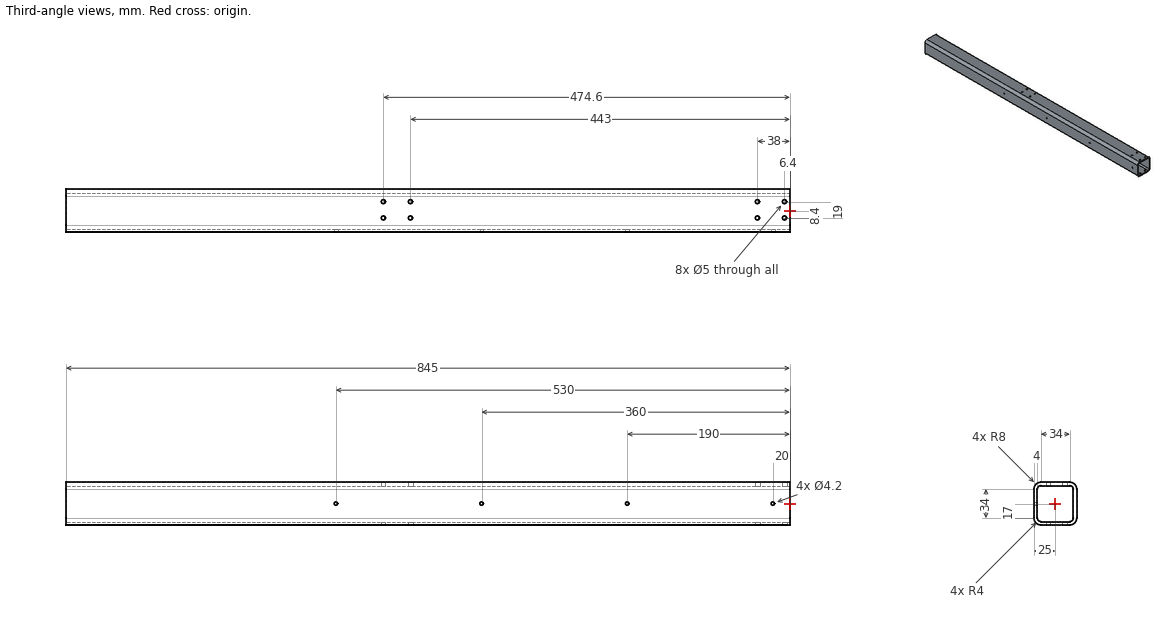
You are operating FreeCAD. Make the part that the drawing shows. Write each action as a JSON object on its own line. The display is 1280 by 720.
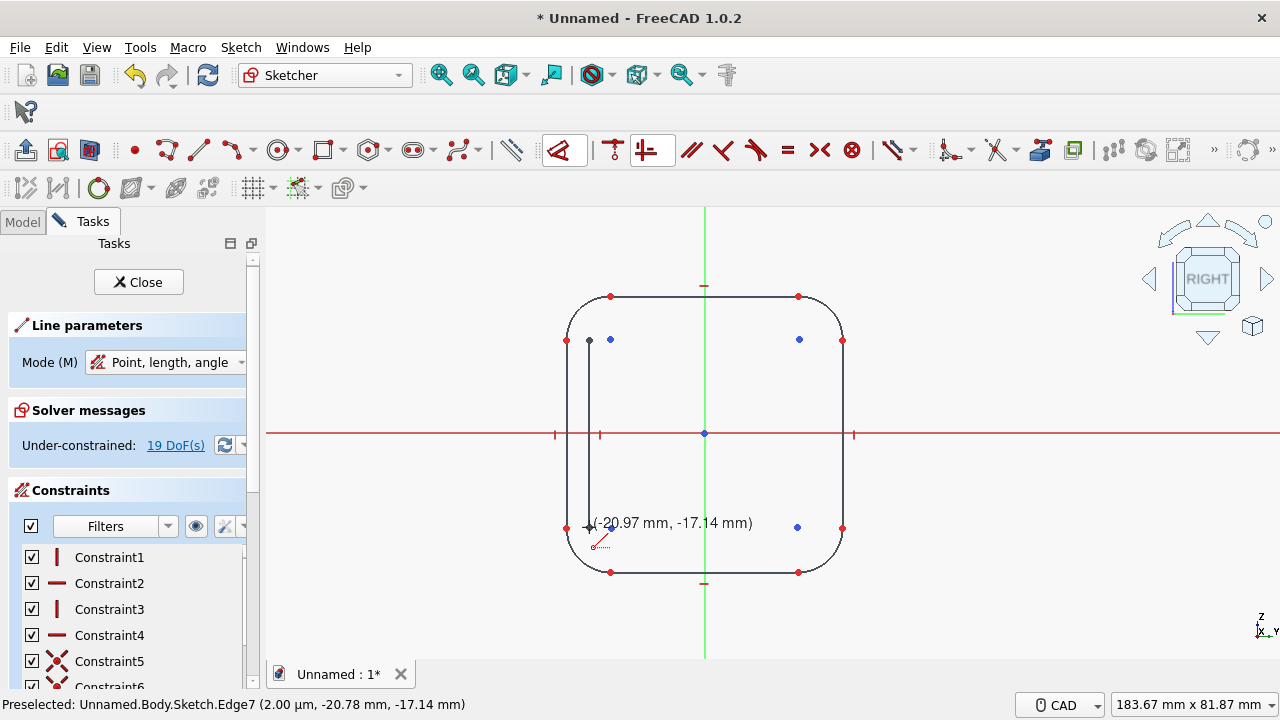
{"action": "left_click", "coordinate": [611, 549]}
{"action": "left_click", "coordinate": [799, 549]}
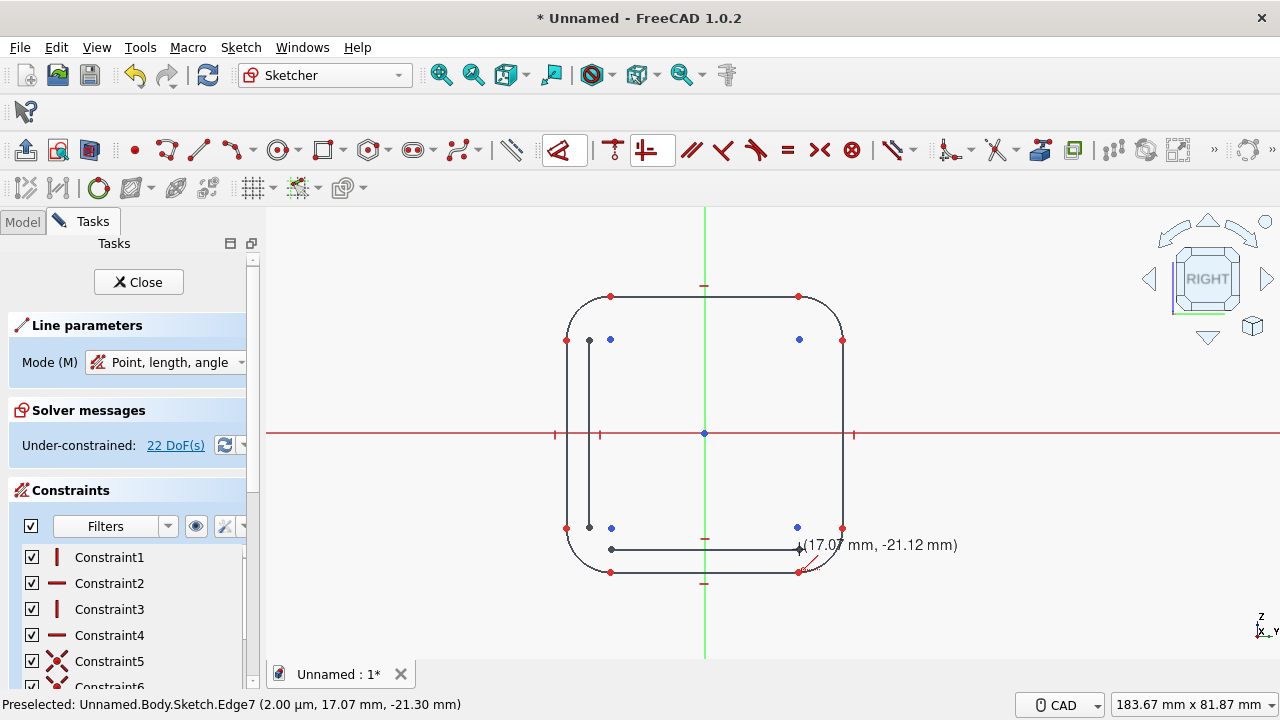
{"action": "left_click", "coordinate": [821, 527]}
{"action": "left_click", "coordinate": [821, 340]}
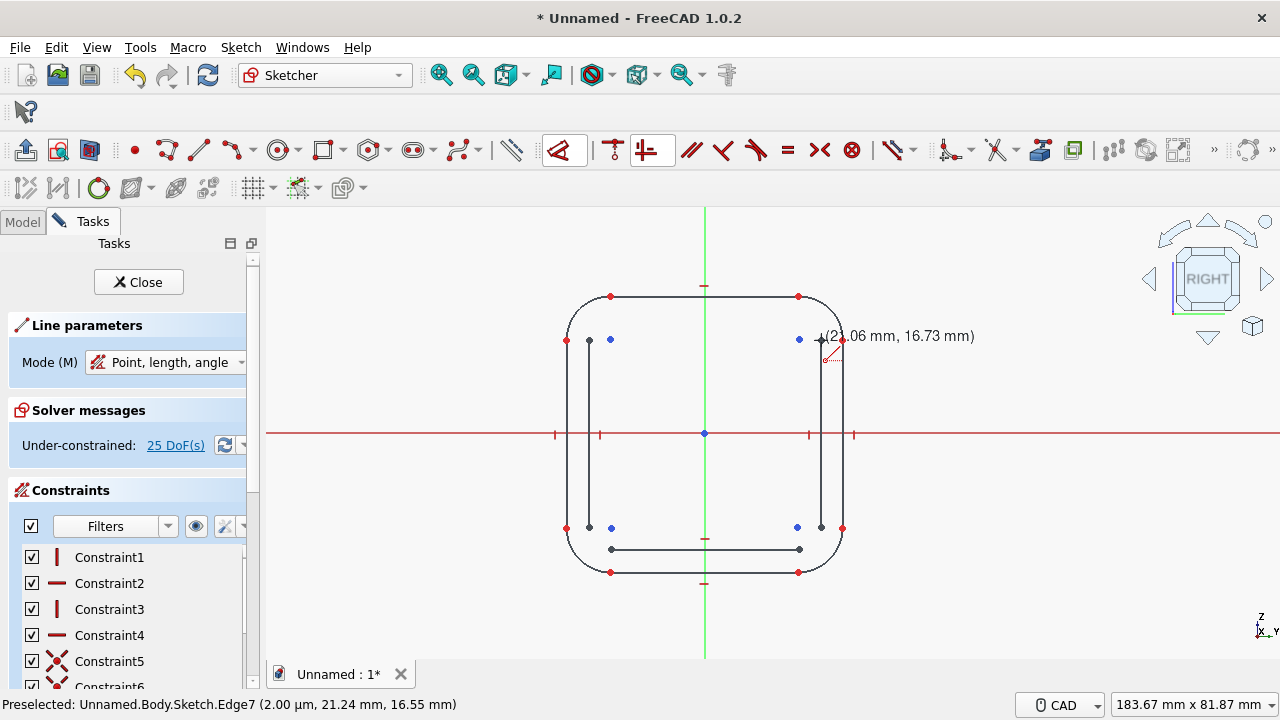
{"action": "left_click", "coordinate": [799, 317]}
{"action": "left_click", "coordinate": [611, 317]}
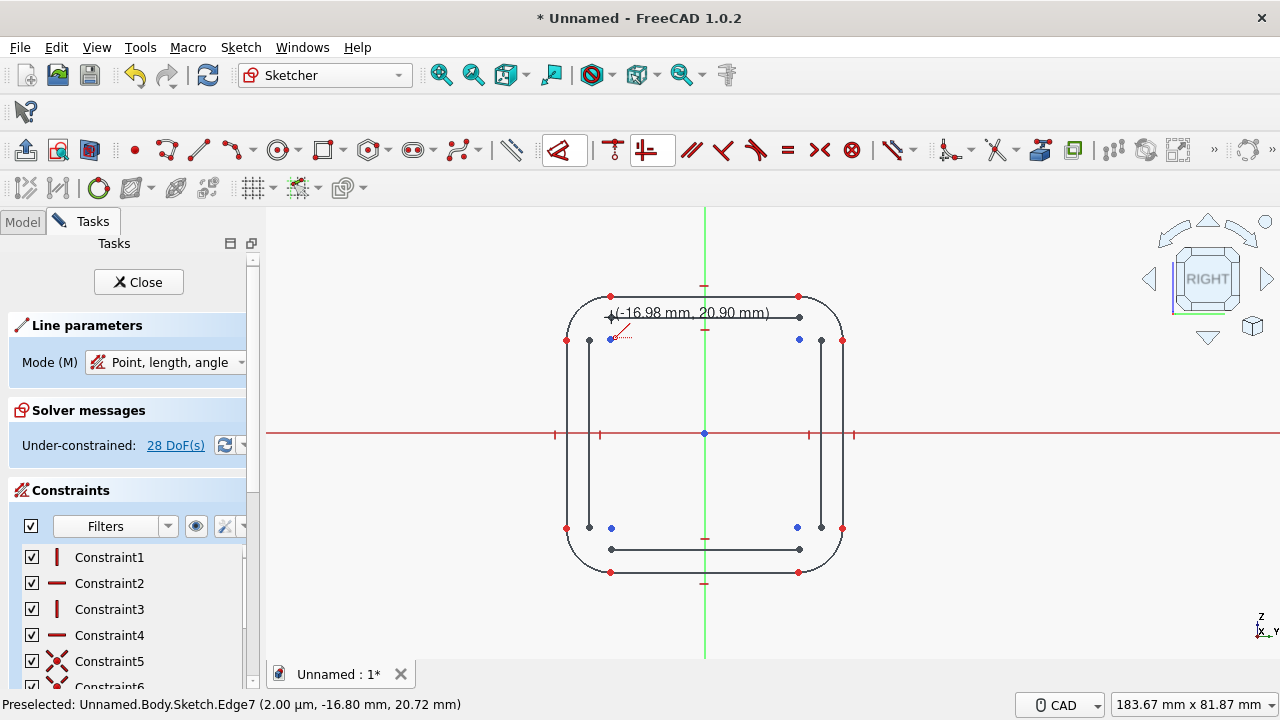
{"action": "left_click", "coordinate": [232, 150]}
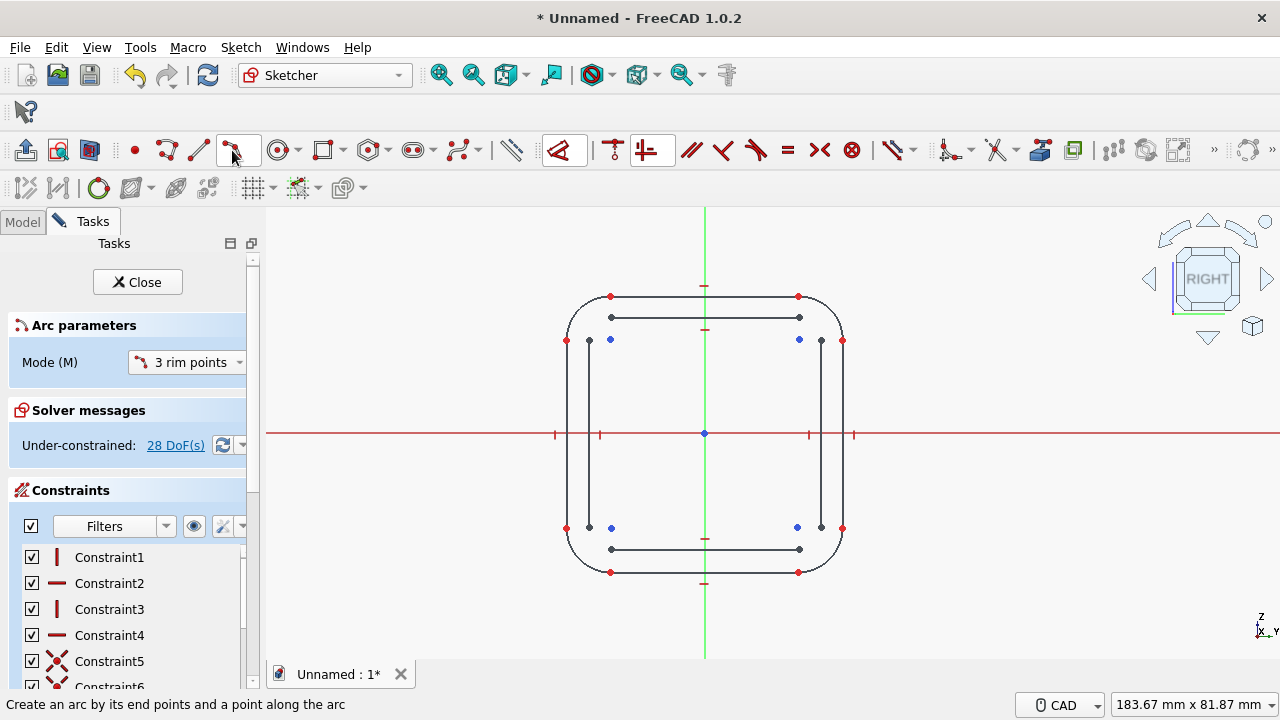
{"action": "left_click", "coordinate": [589, 528]}
{"action": "left_click", "coordinate": [611, 550]}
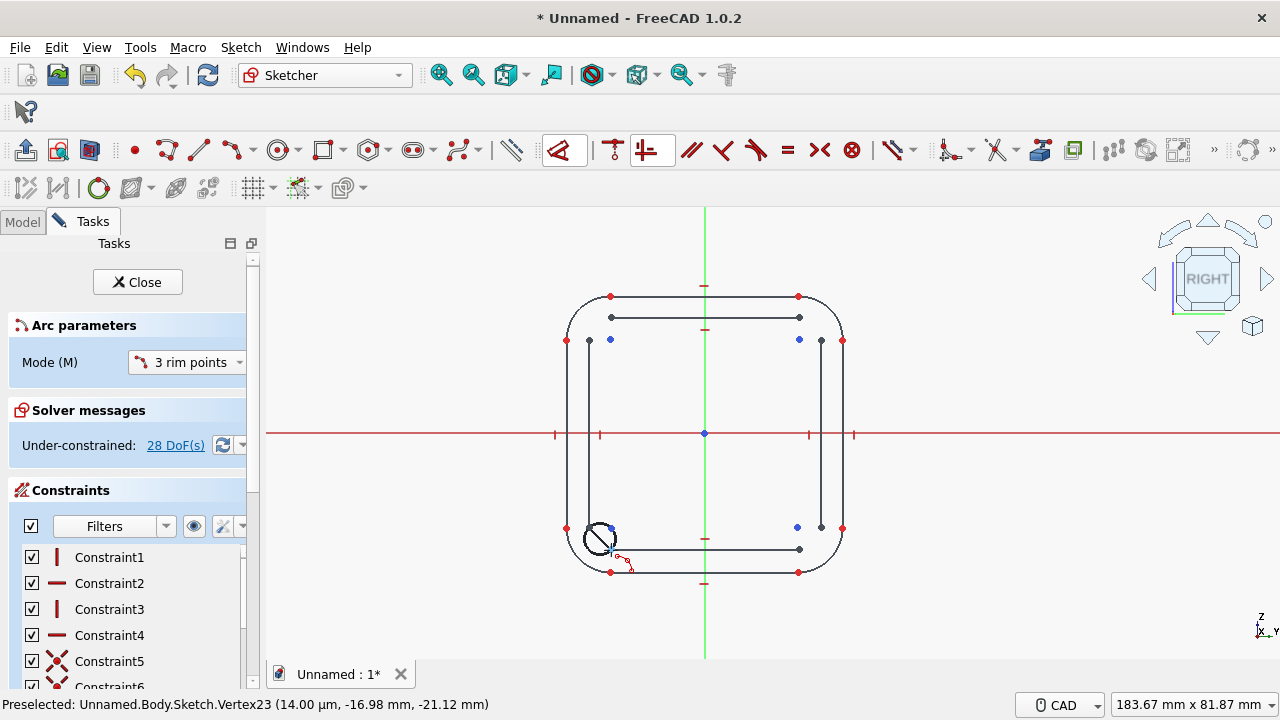
{"action": "scroll", "coordinate": [595, 543], "scroll_direction": "up", "scroll_amount": 5}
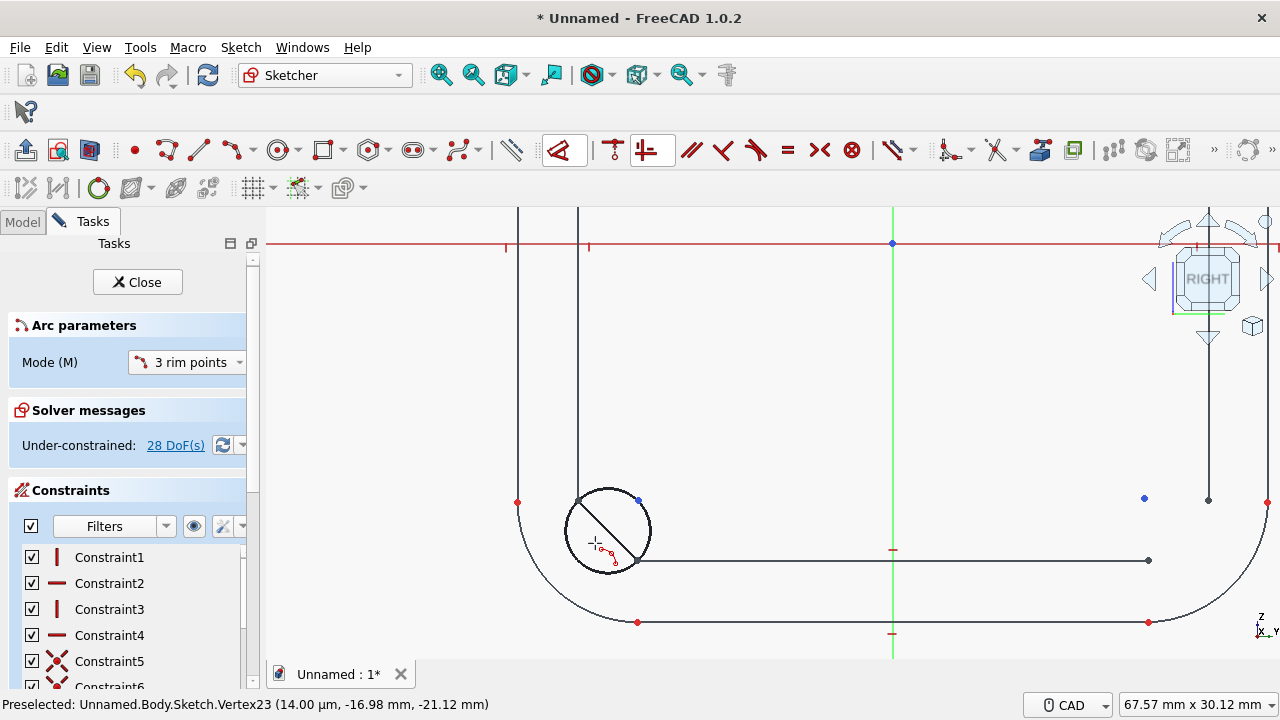
{"action": "left_click", "coordinate": [595, 541]}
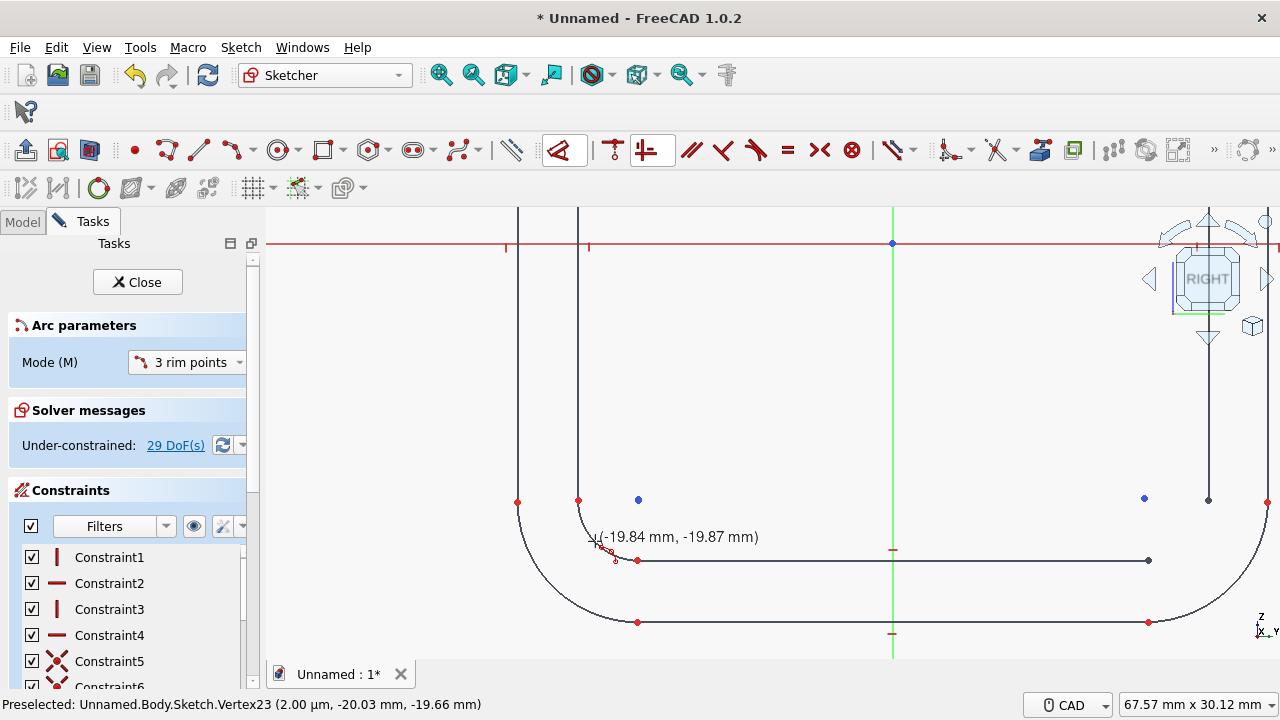
{"action": "scroll", "coordinate": [595, 543], "scroll_direction": "down", "scroll_amount": 5}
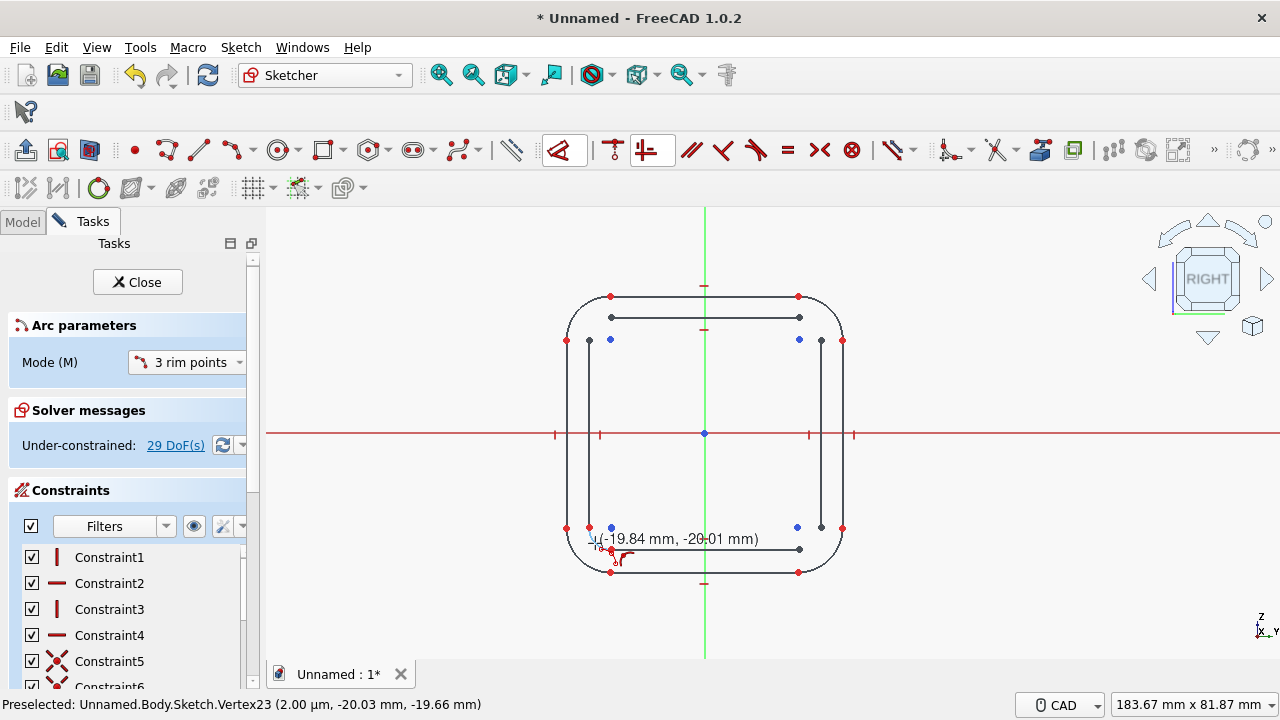
{"action": "left_click", "coordinate": [799, 550]}
{"action": "left_click", "coordinate": [821, 528]}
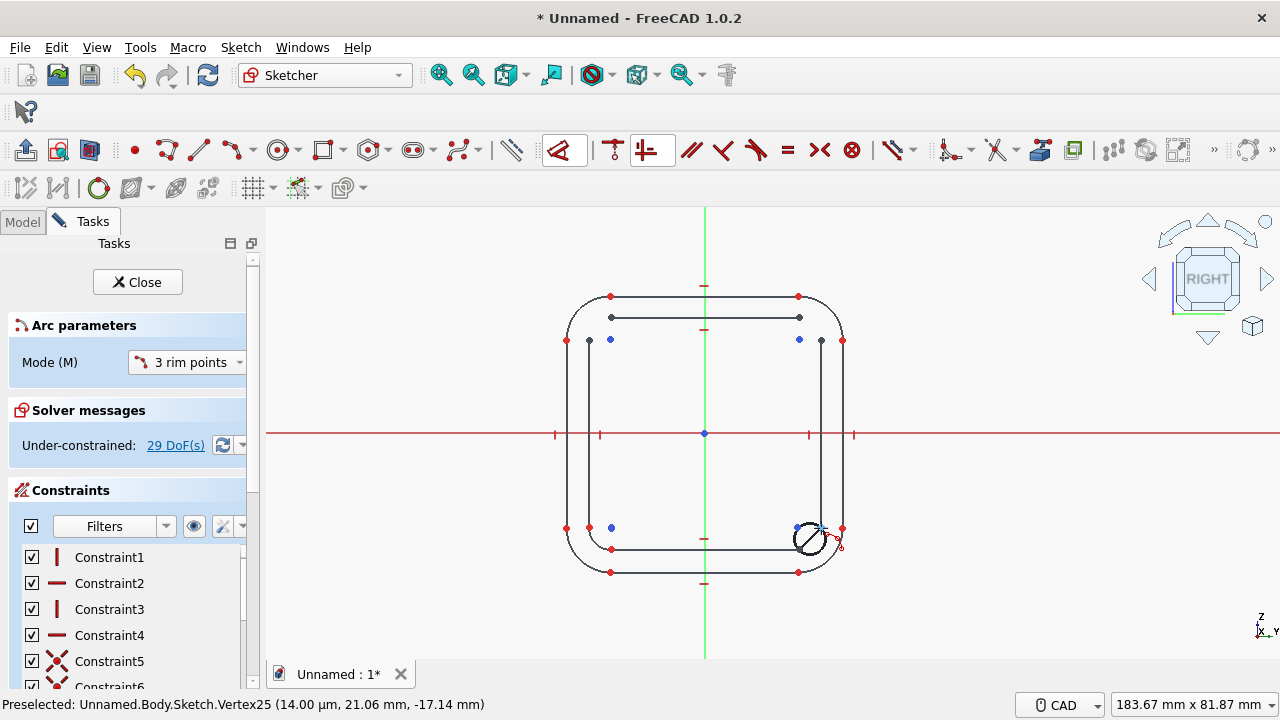
{"action": "scroll", "coordinate": [814, 543], "scroll_direction": "up", "scroll_amount": 5}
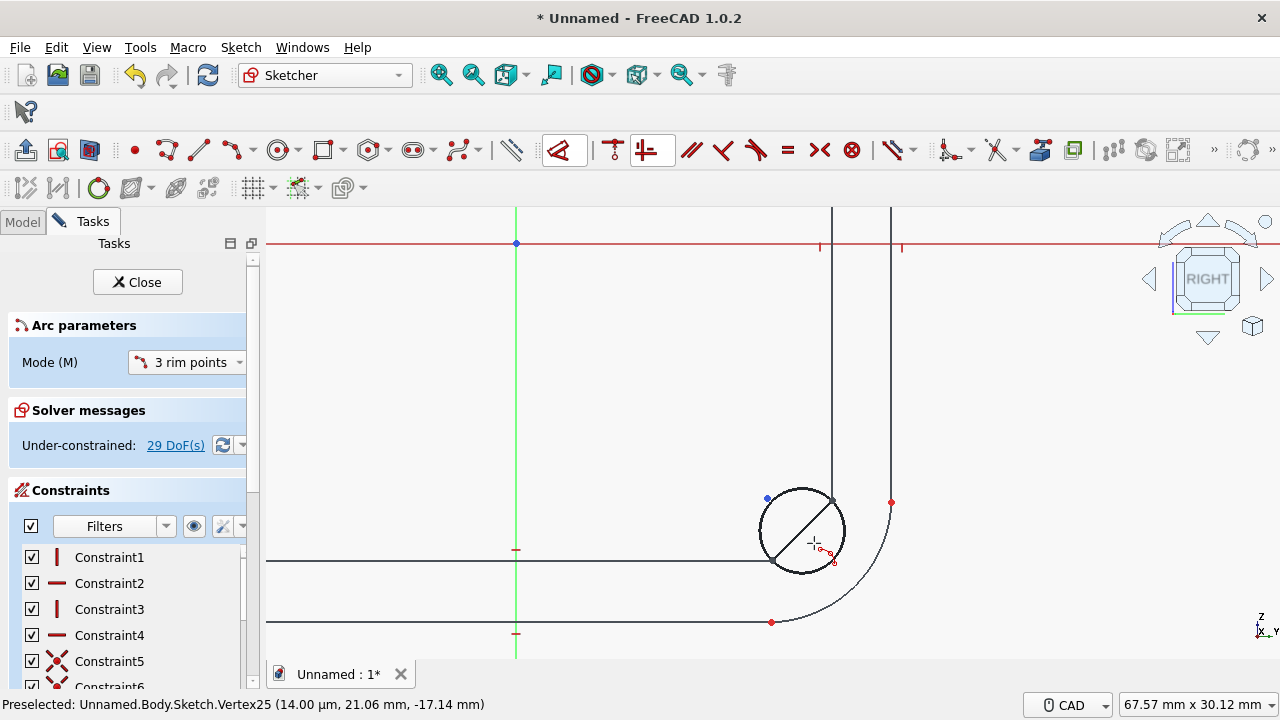
{"action": "left_click", "coordinate": [814, 541]}